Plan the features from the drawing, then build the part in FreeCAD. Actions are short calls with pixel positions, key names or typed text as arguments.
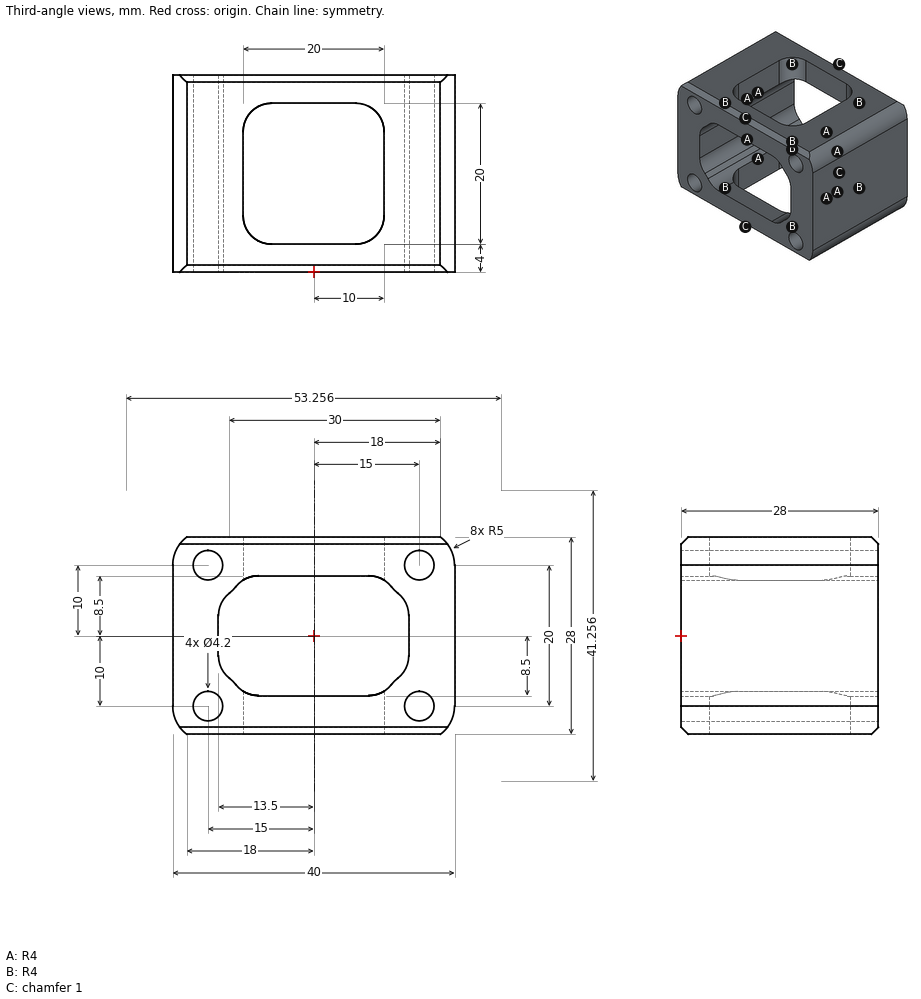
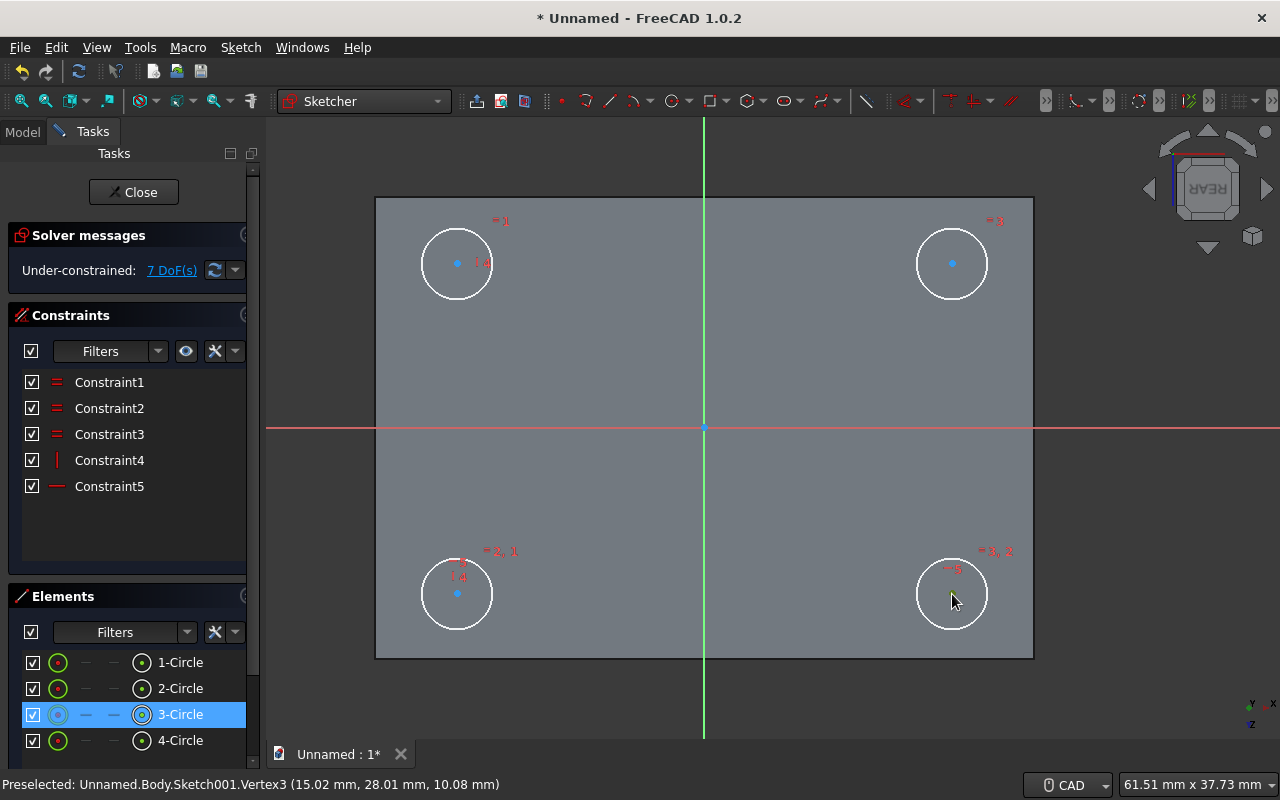
click(952, 264)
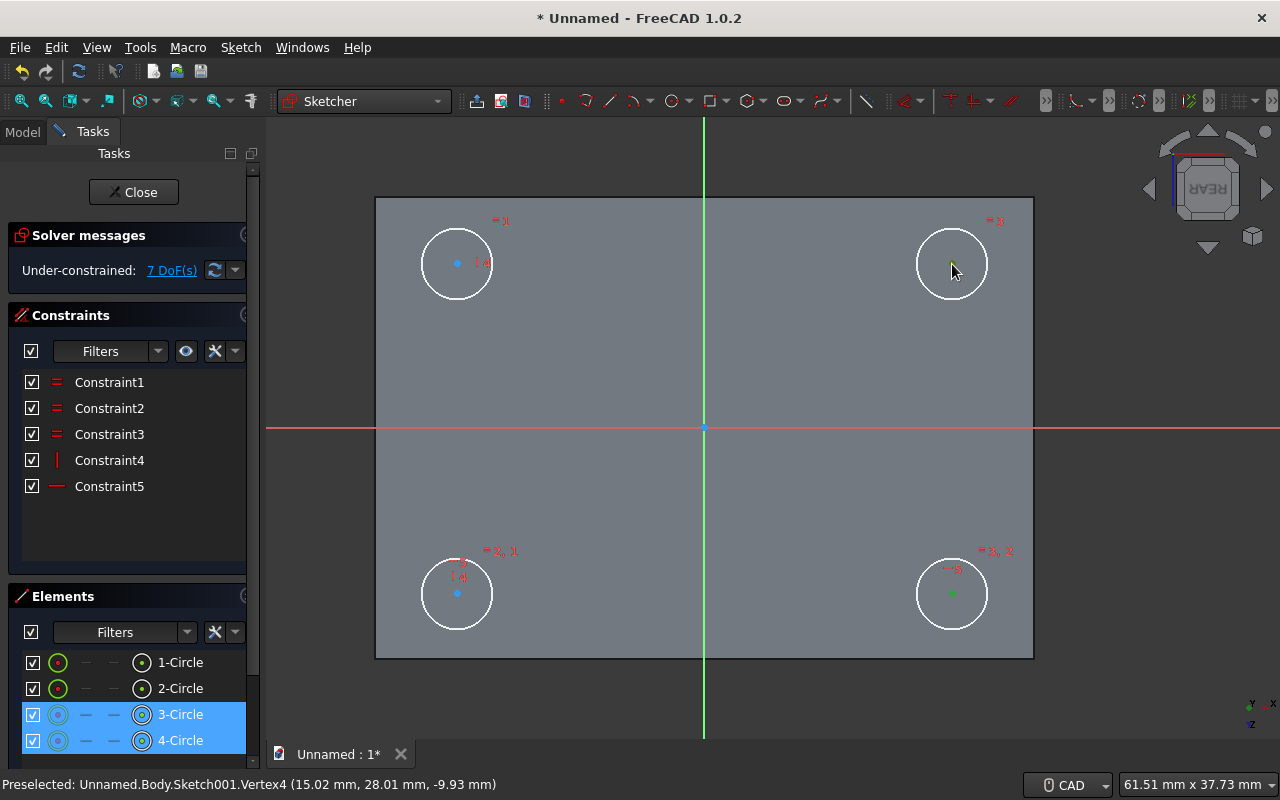
click(992, 102)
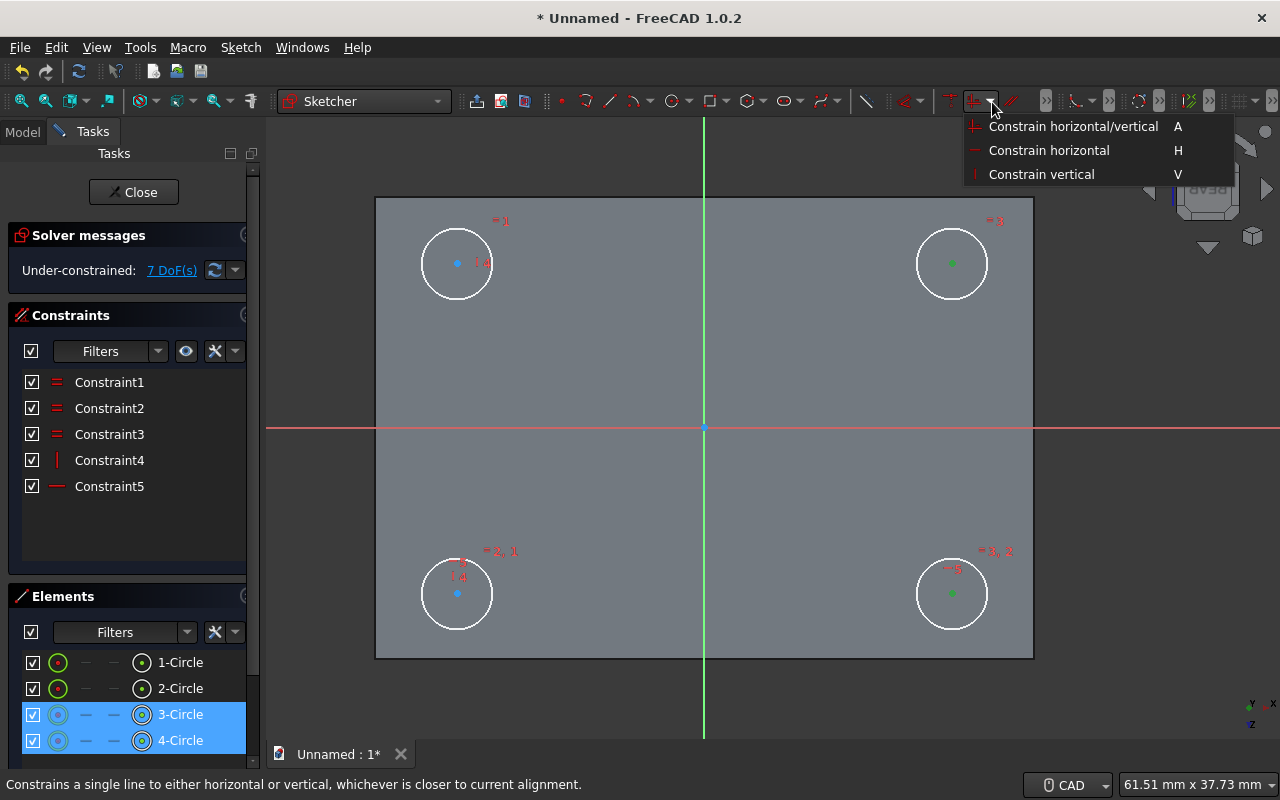
click(1099, 174)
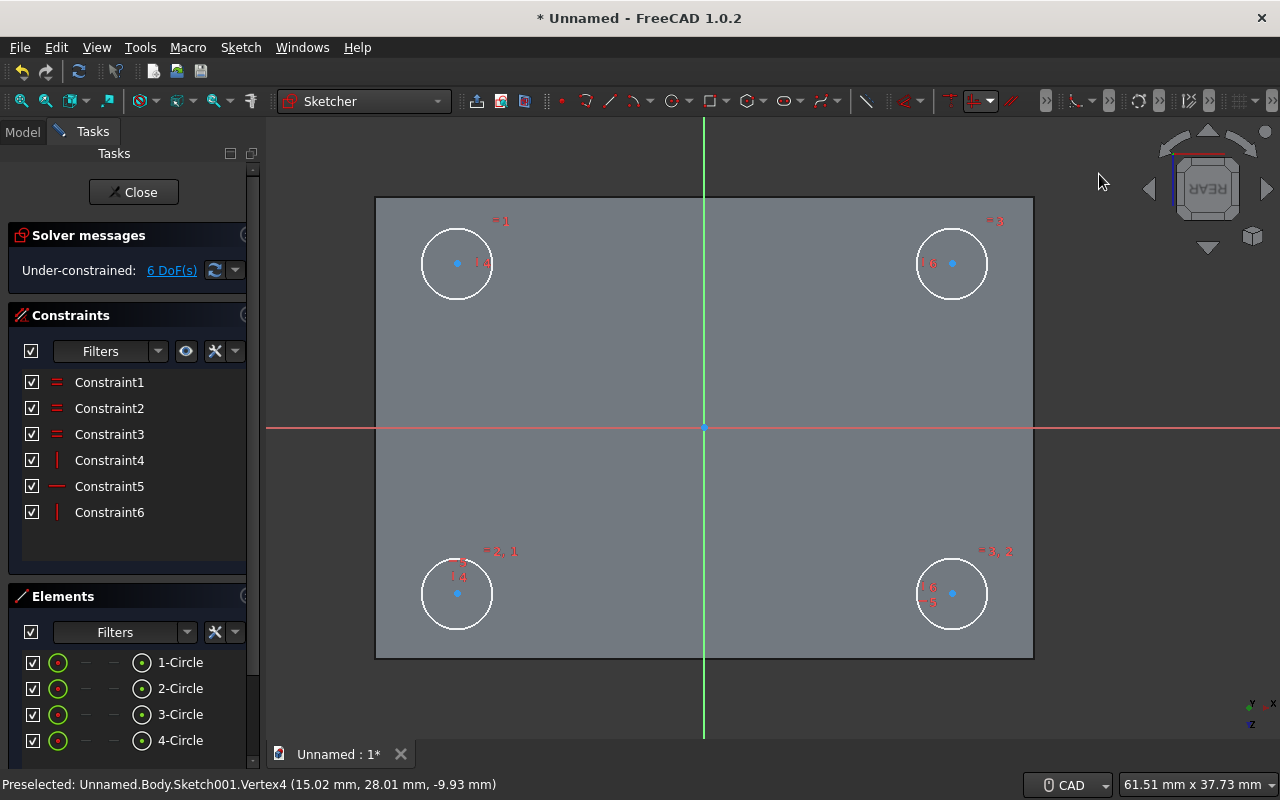
click(457, 264)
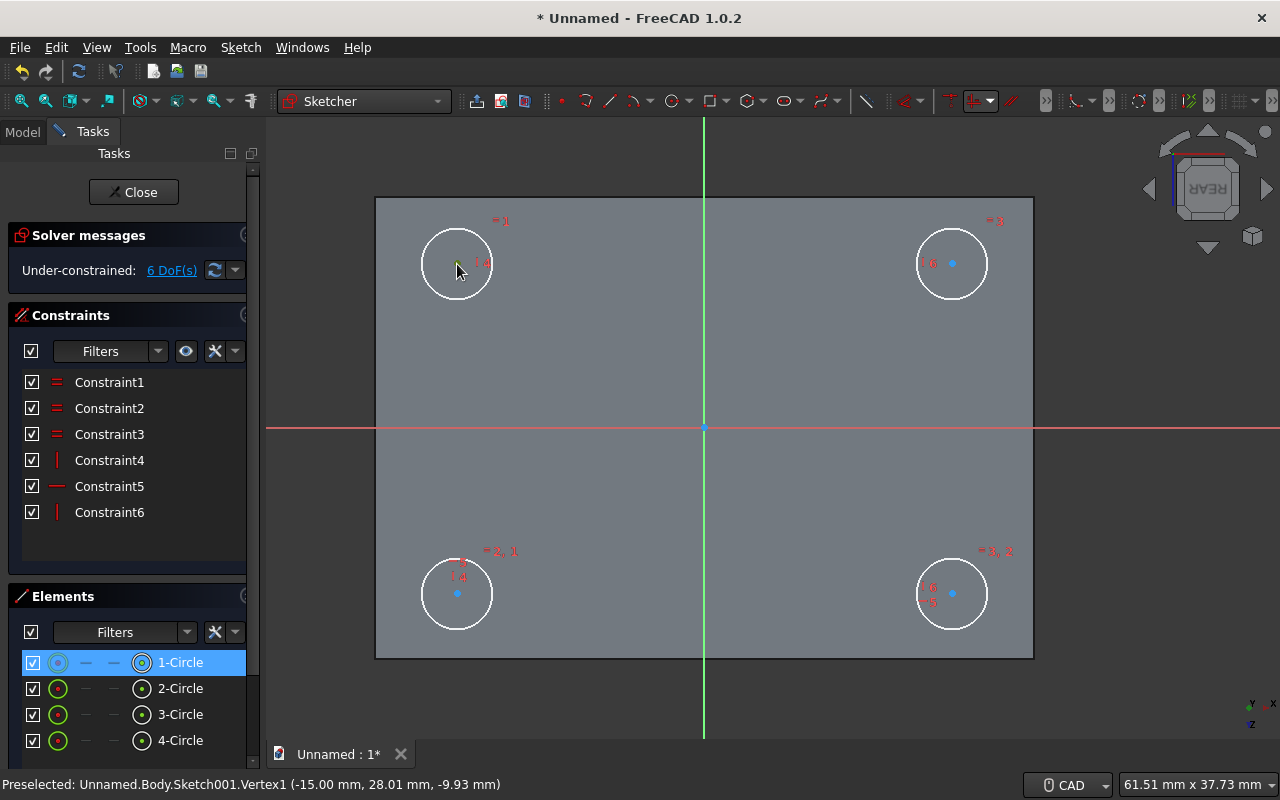
click(952, 264)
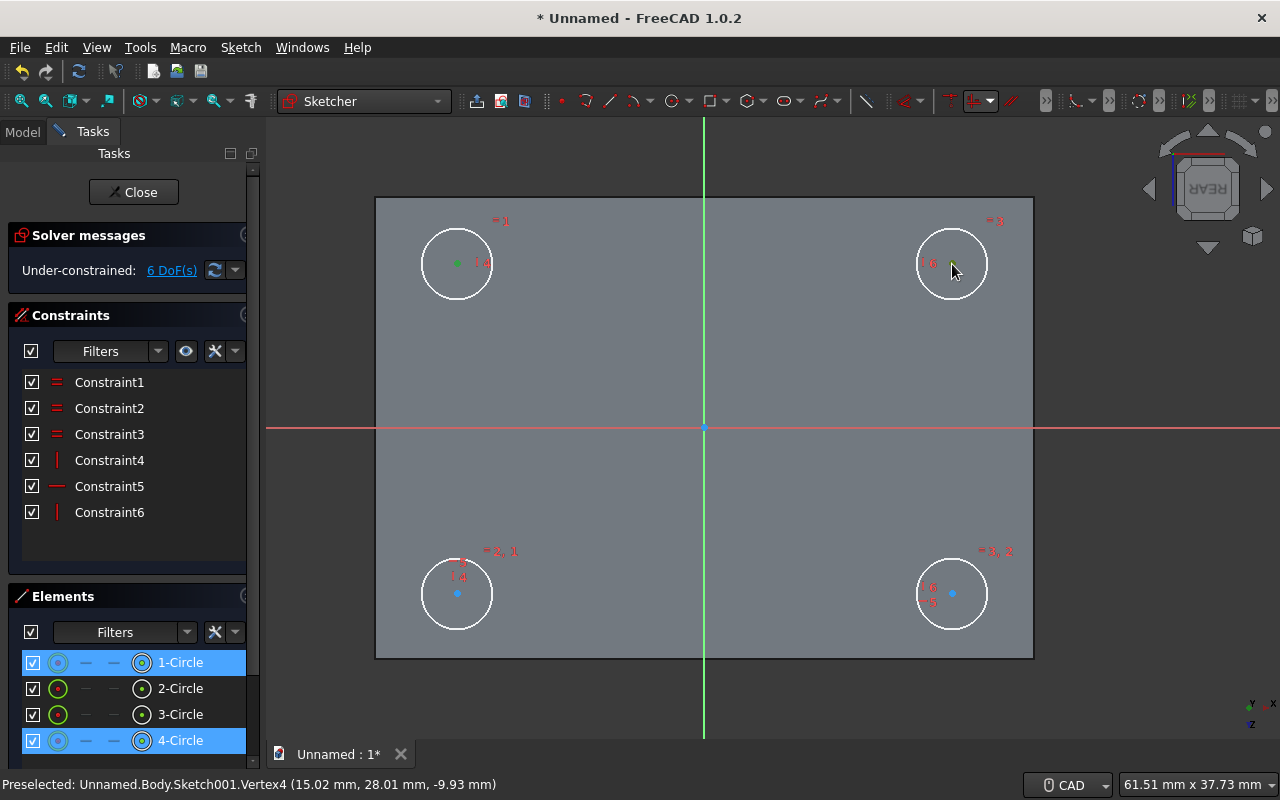
key(h)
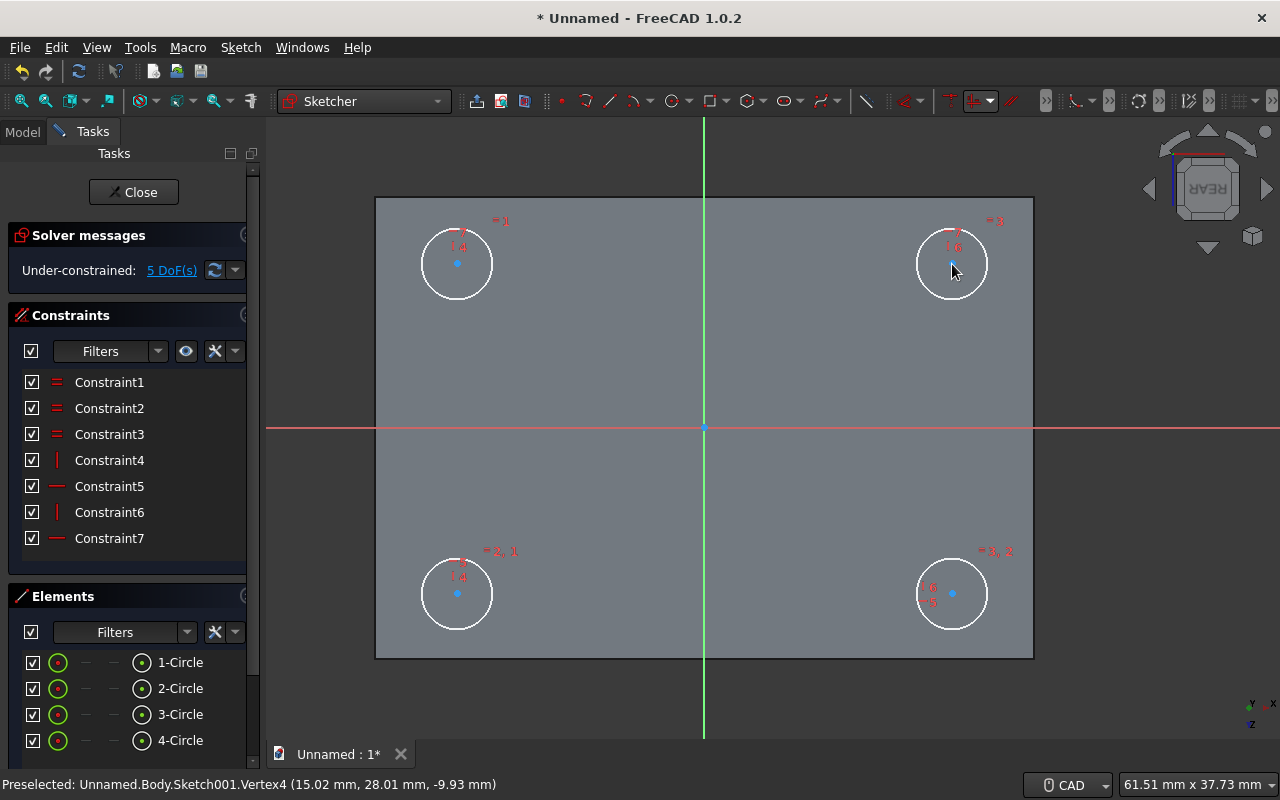
click(482, 239)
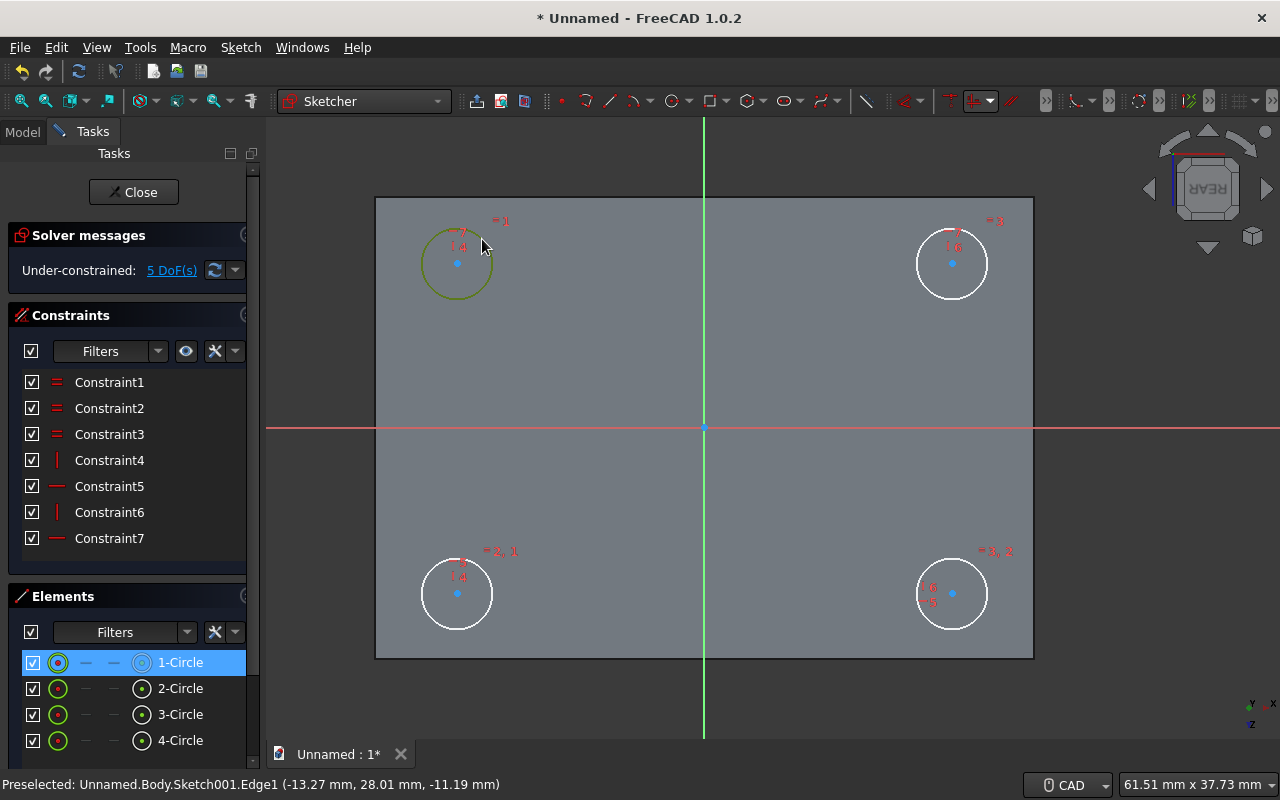
click(922, 102)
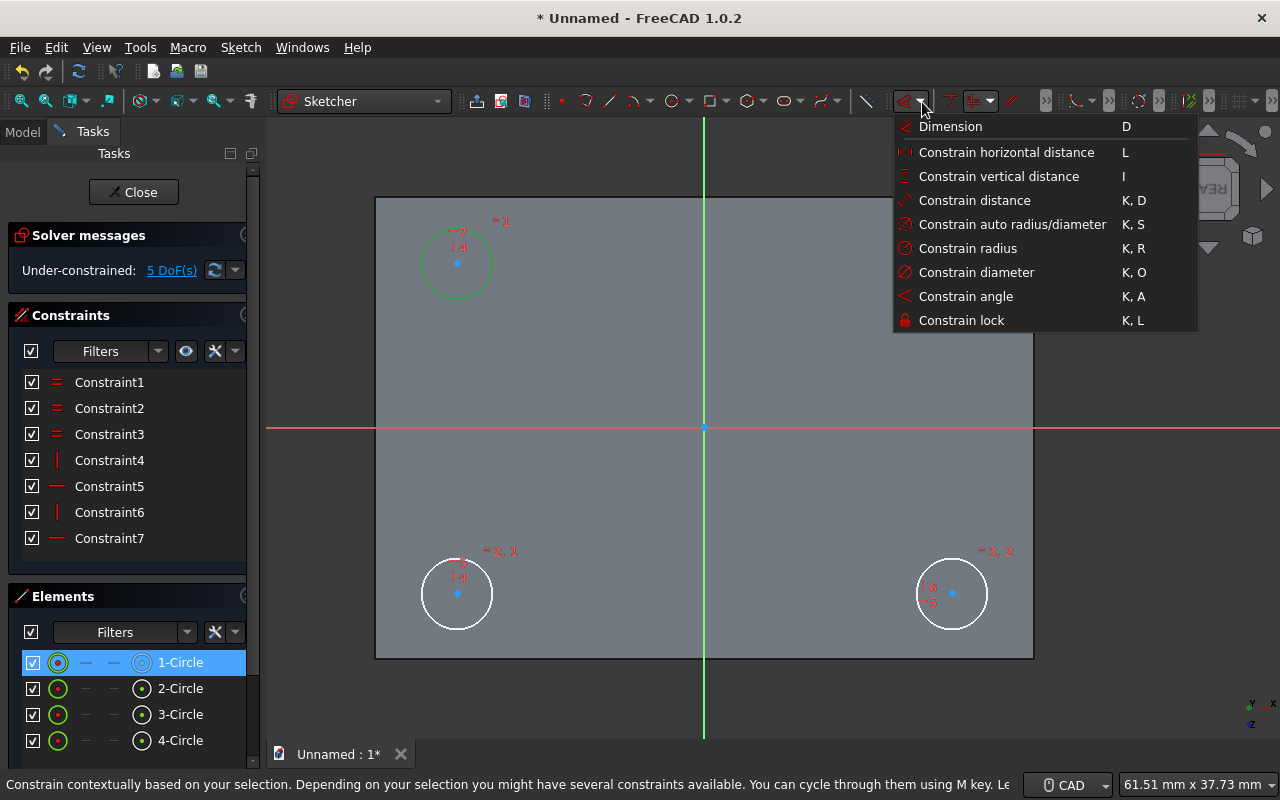
click(1046, 272)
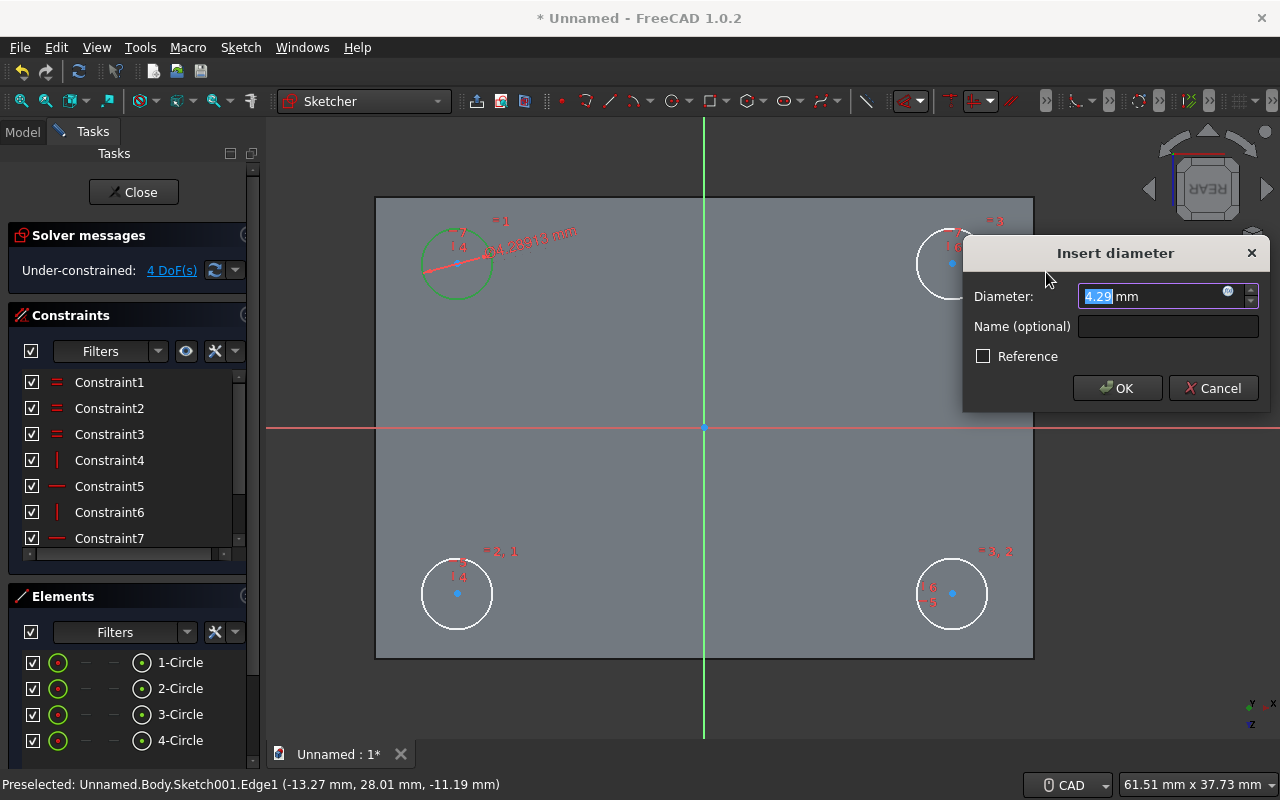
text(4.2)
key(Return)